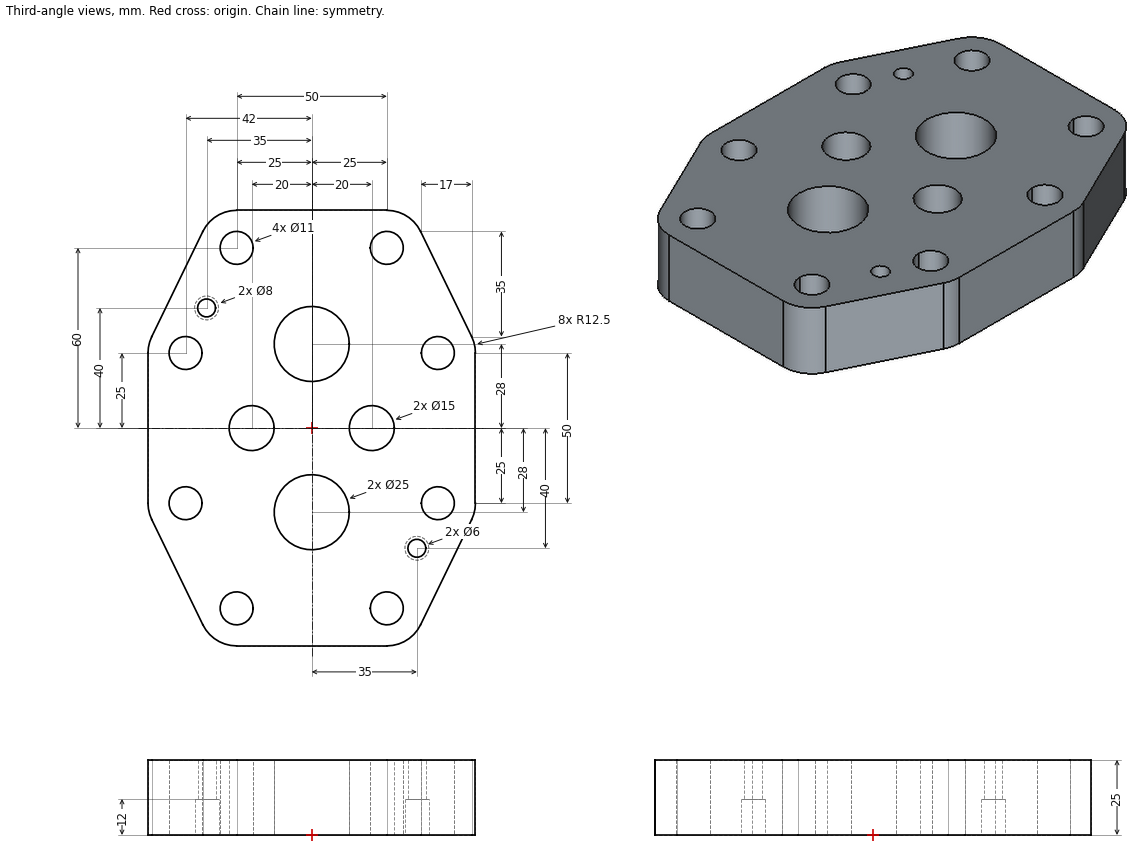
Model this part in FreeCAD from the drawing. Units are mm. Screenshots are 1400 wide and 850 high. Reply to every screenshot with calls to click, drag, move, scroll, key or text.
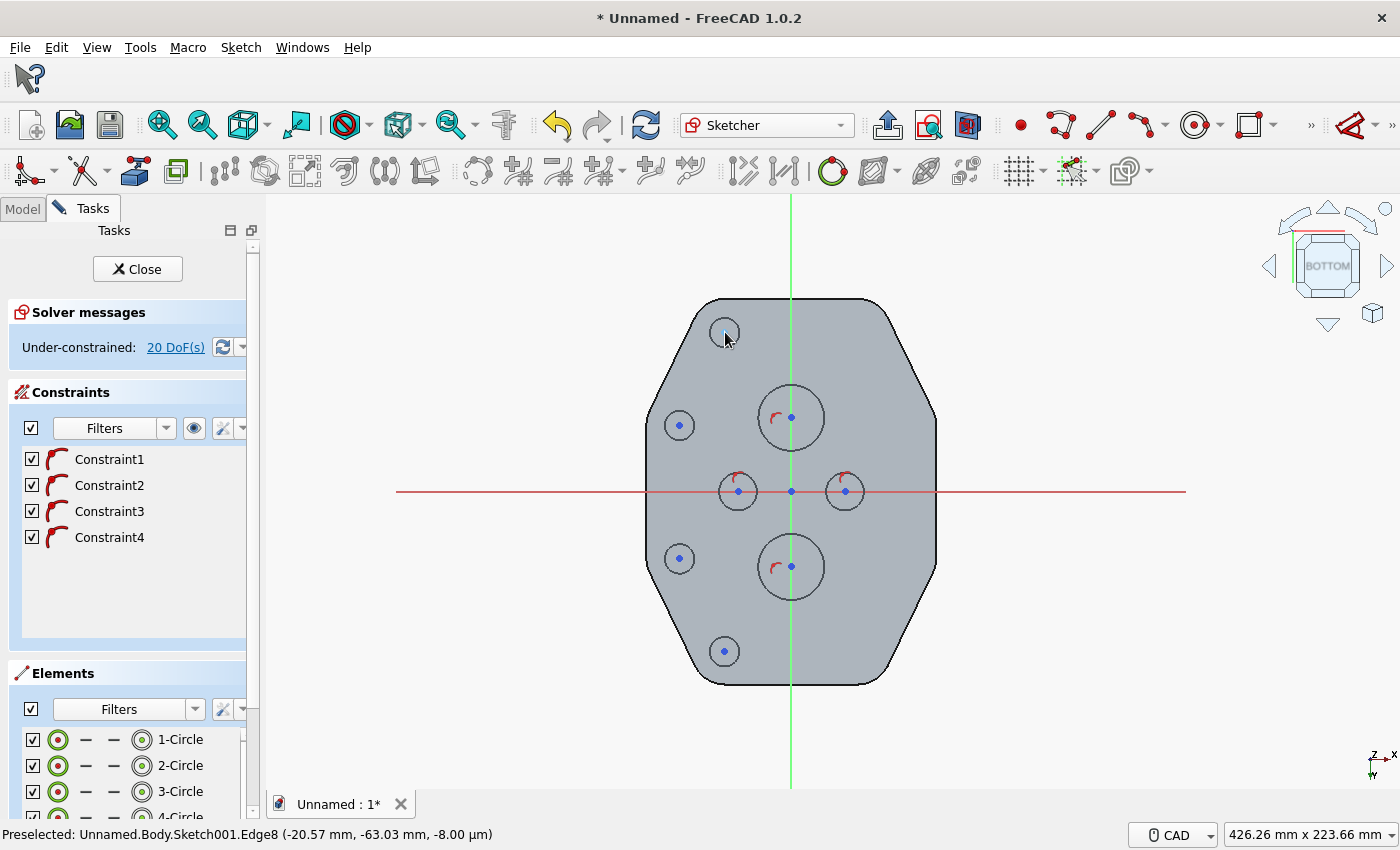
click(735, 641)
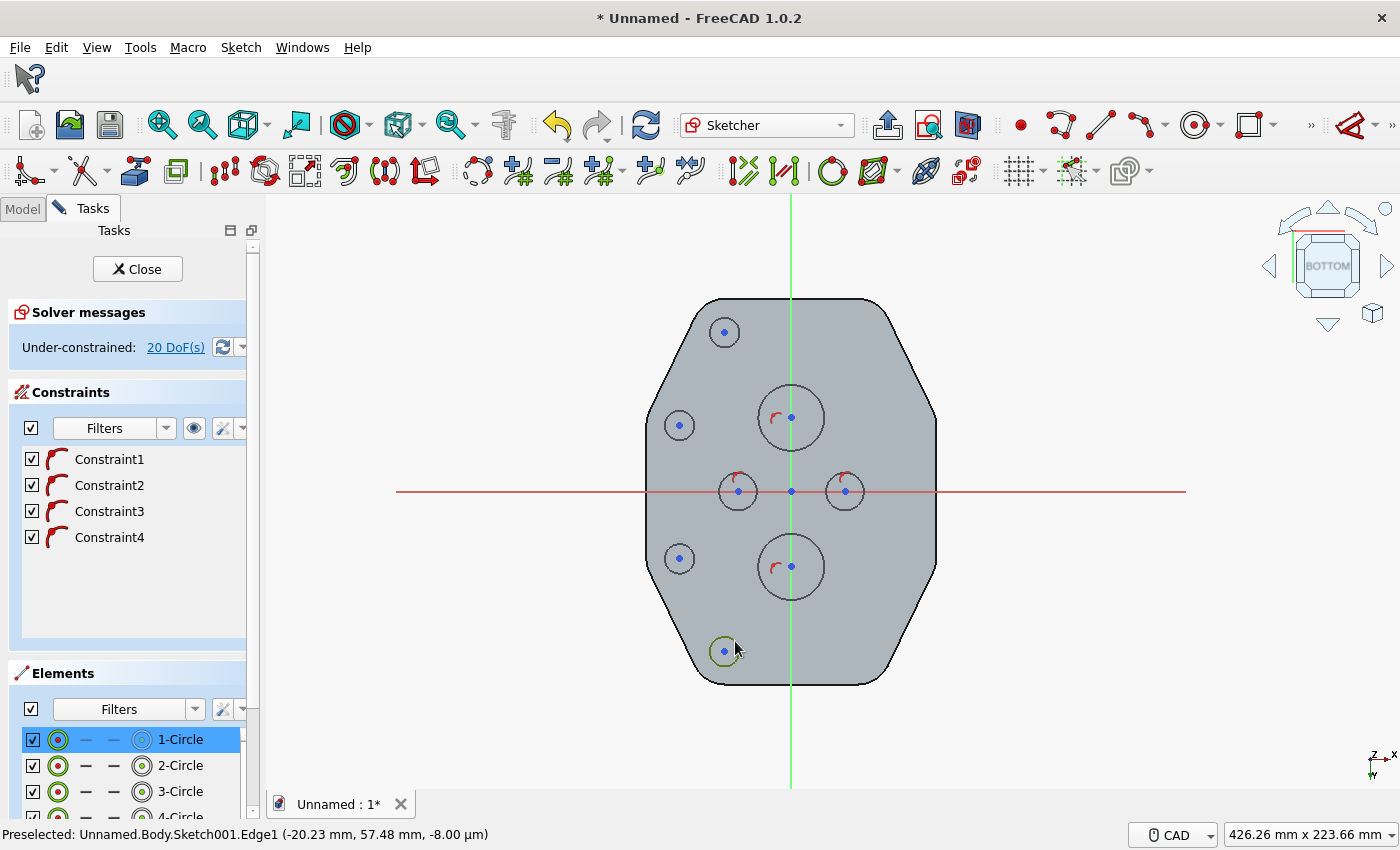
click(690, 548)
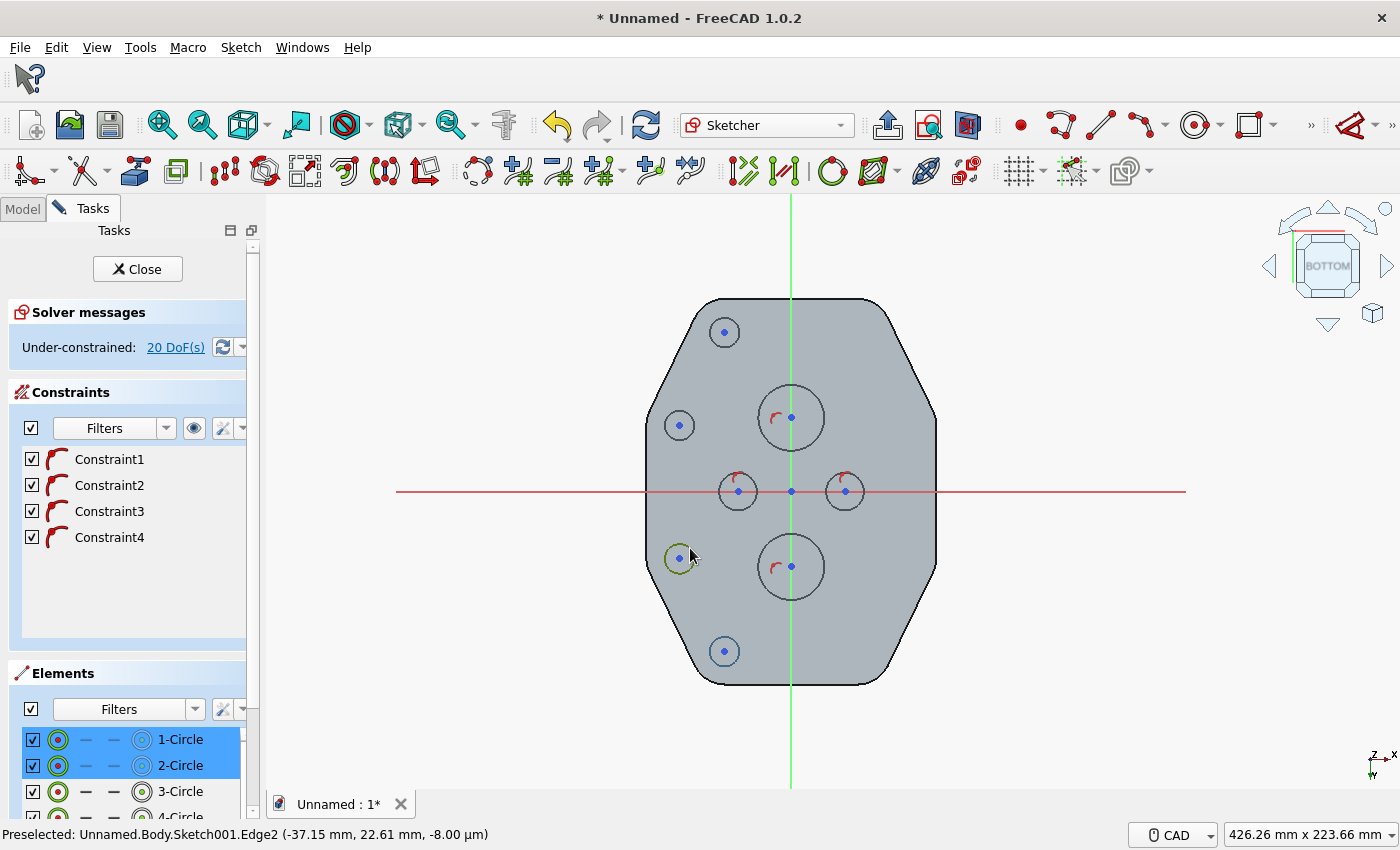
click(690, 415)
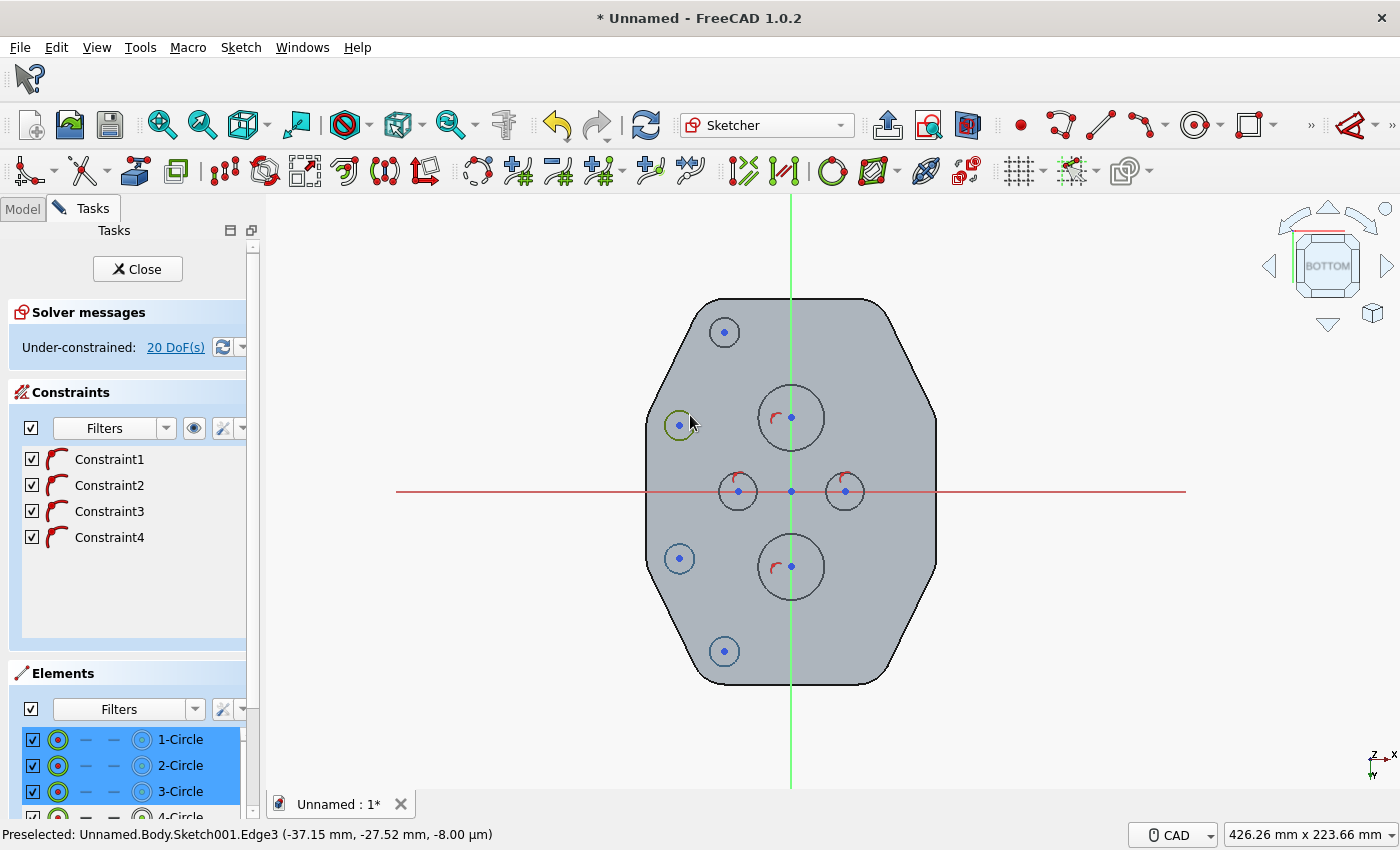
click(735, 322)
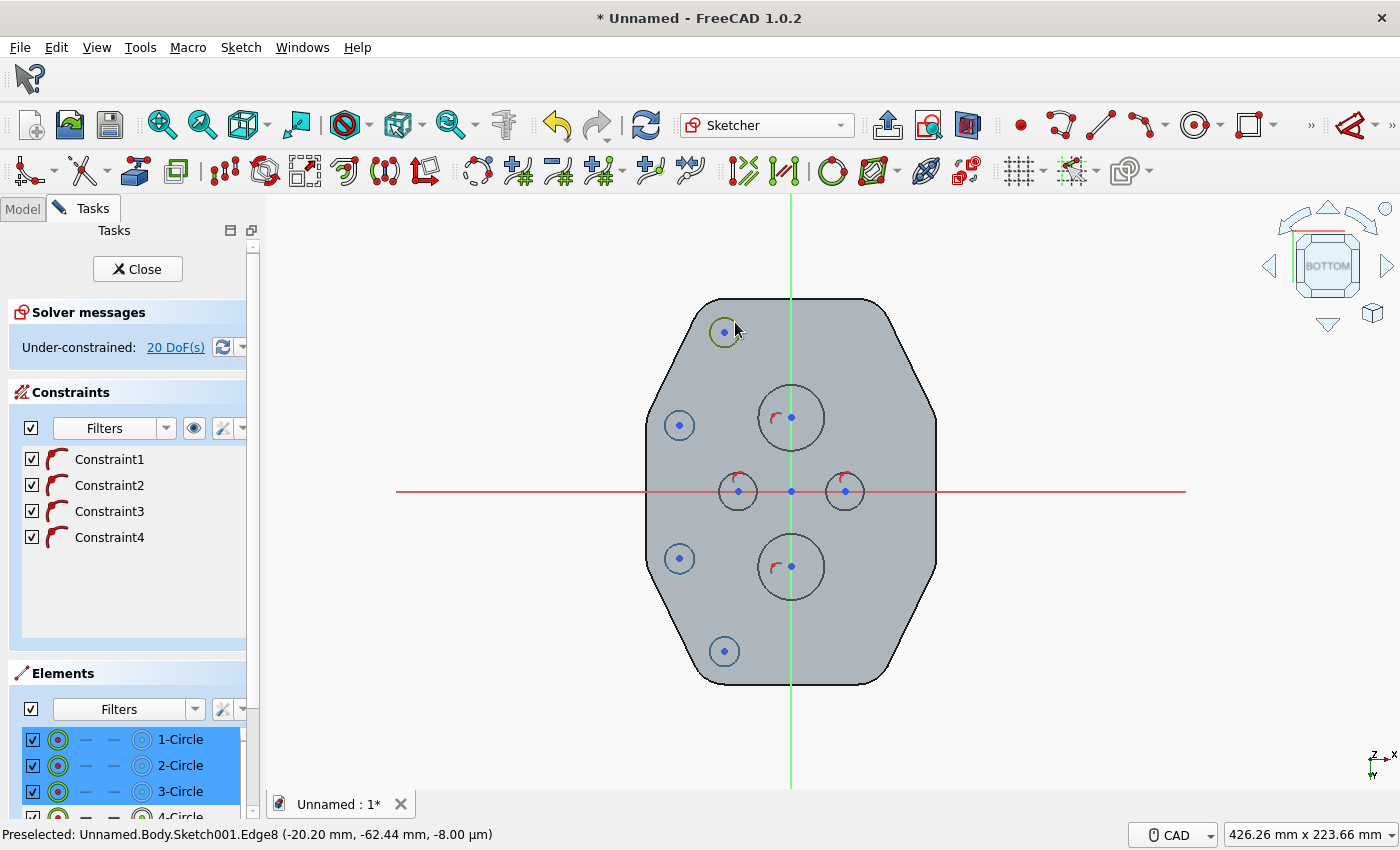
key(e)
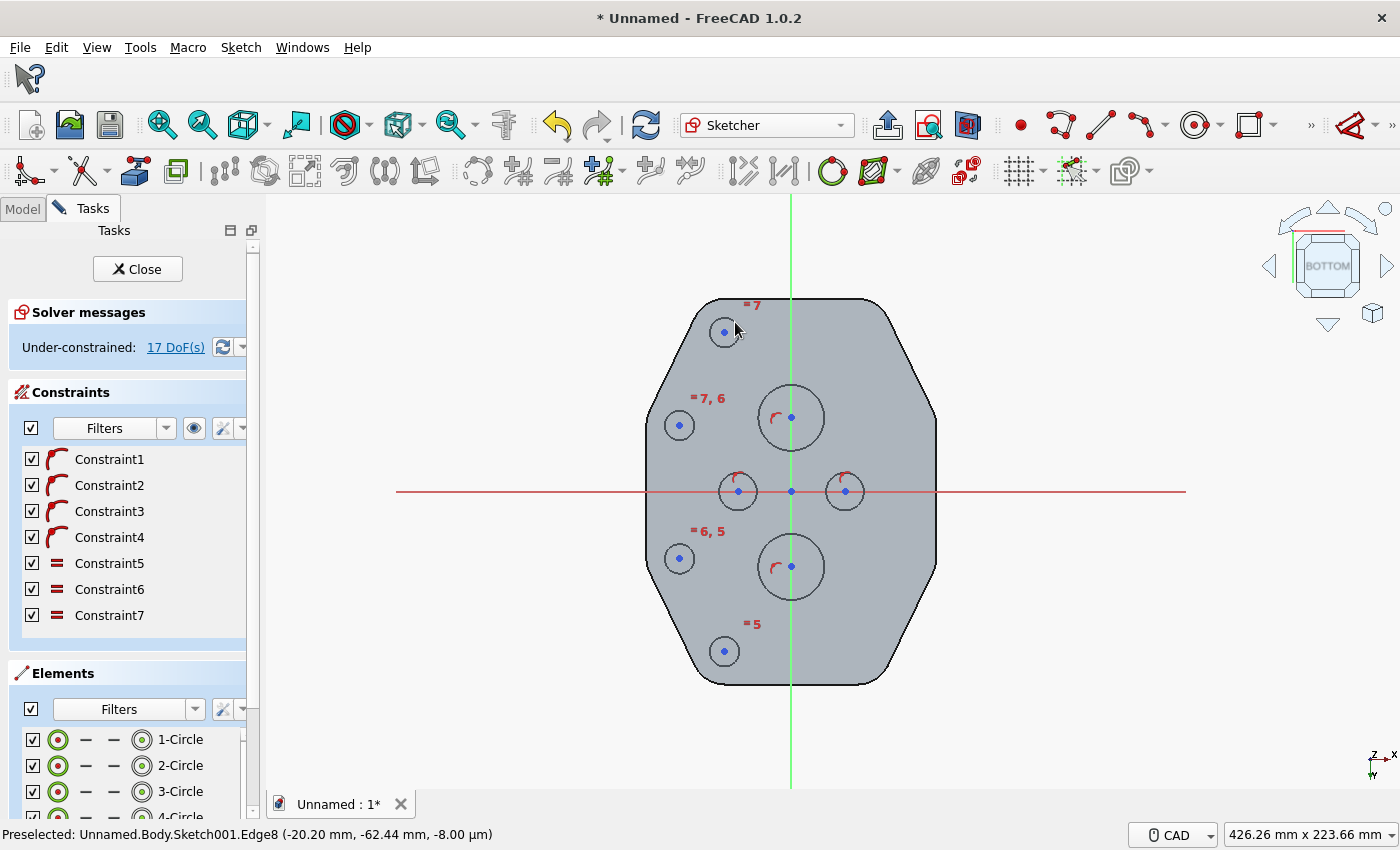
click(858, 478)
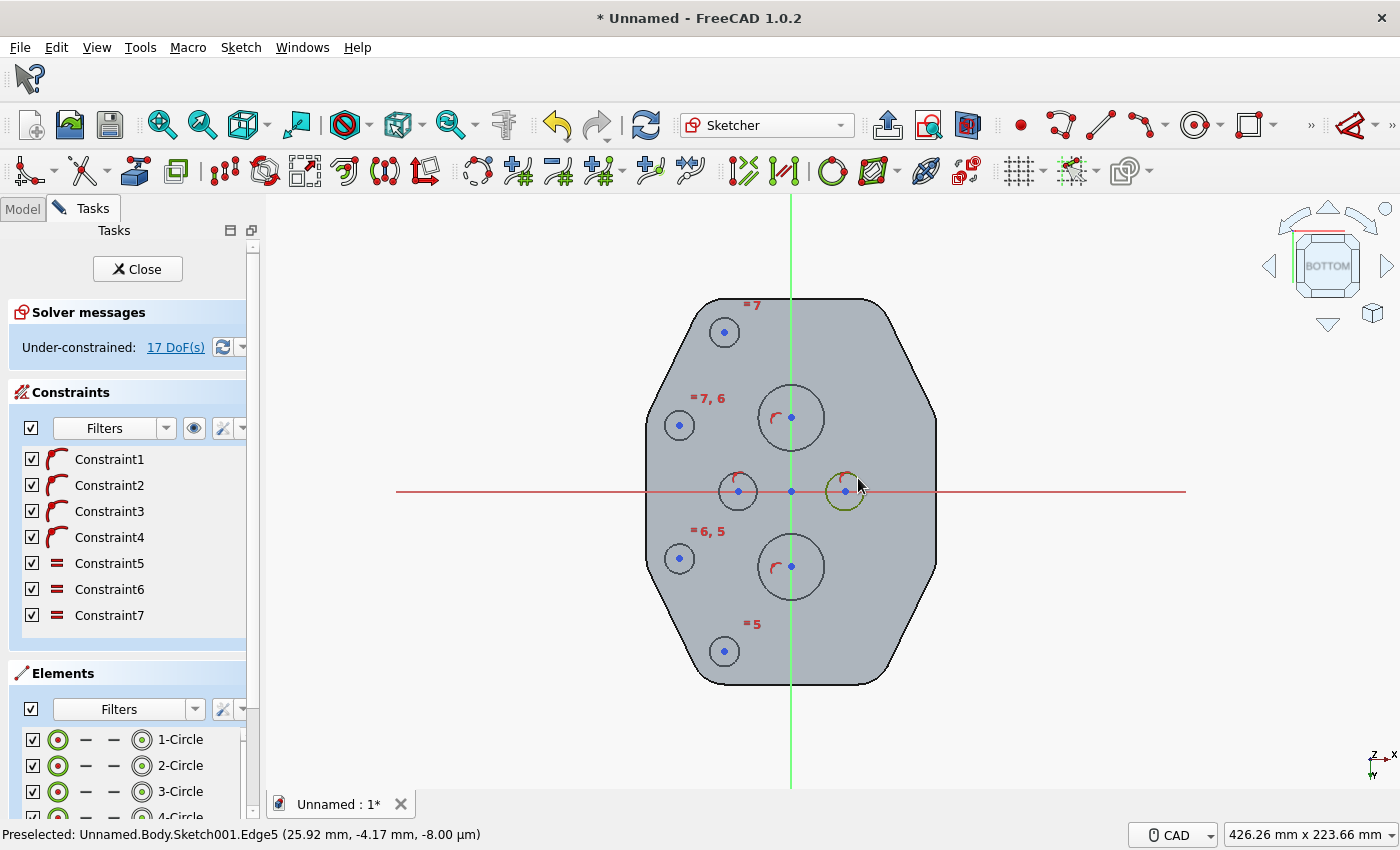
click(751, 478)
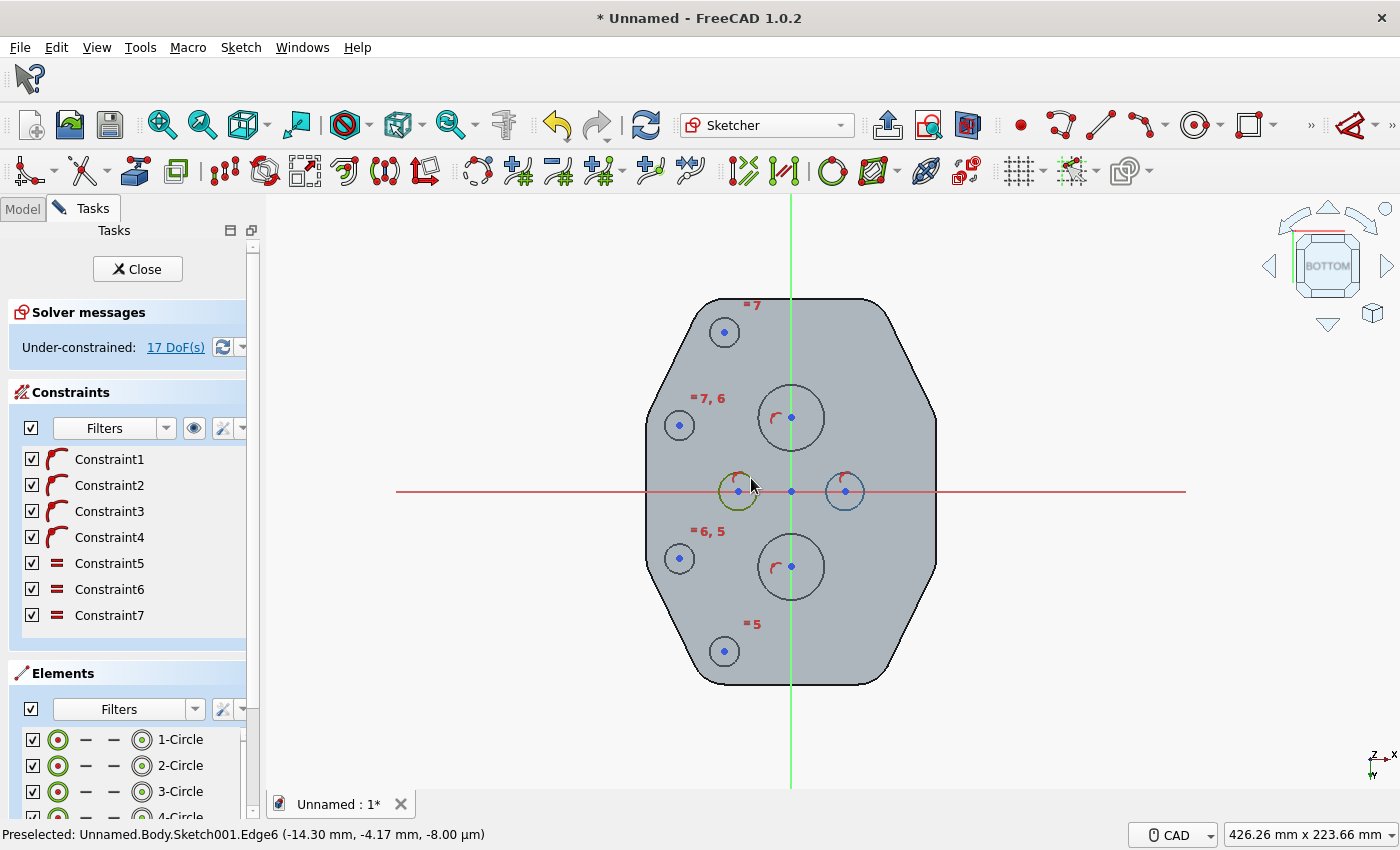
key(e)